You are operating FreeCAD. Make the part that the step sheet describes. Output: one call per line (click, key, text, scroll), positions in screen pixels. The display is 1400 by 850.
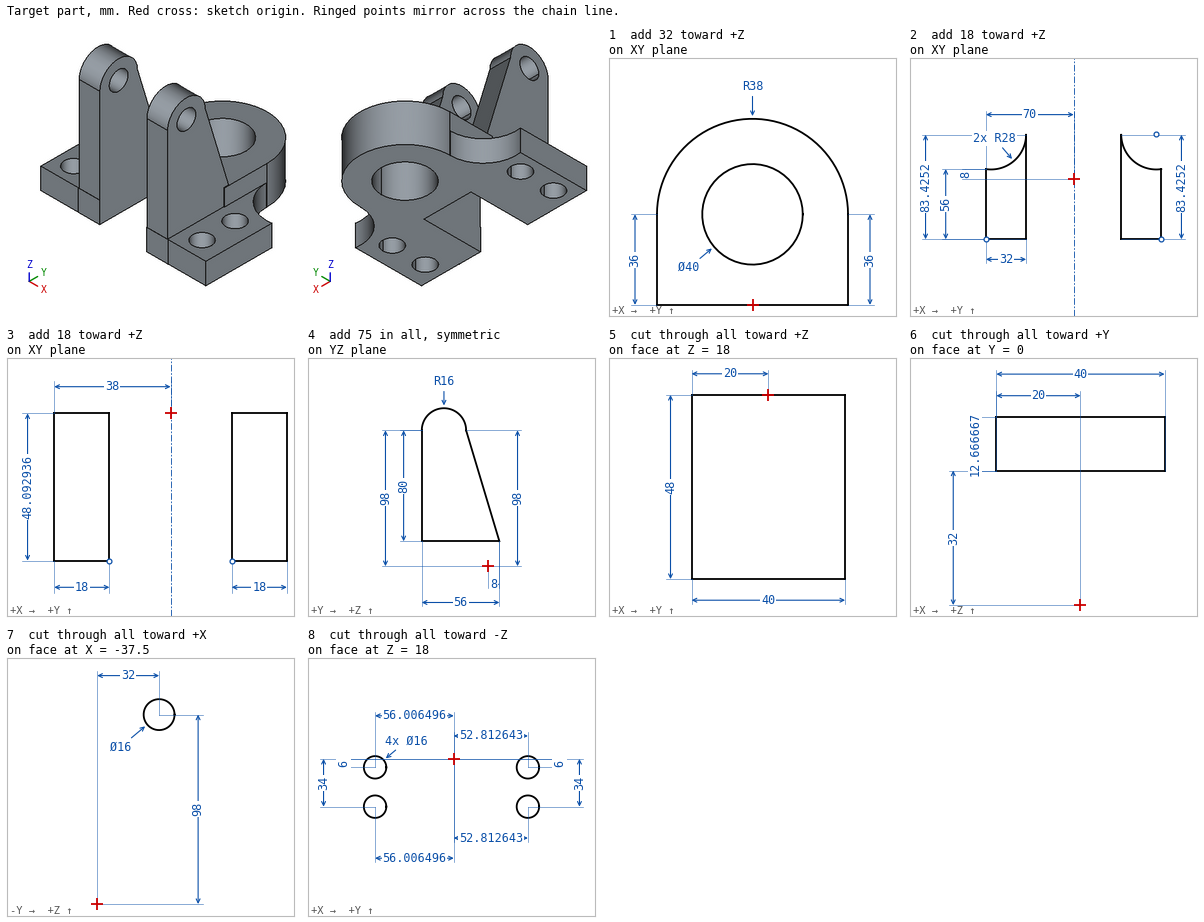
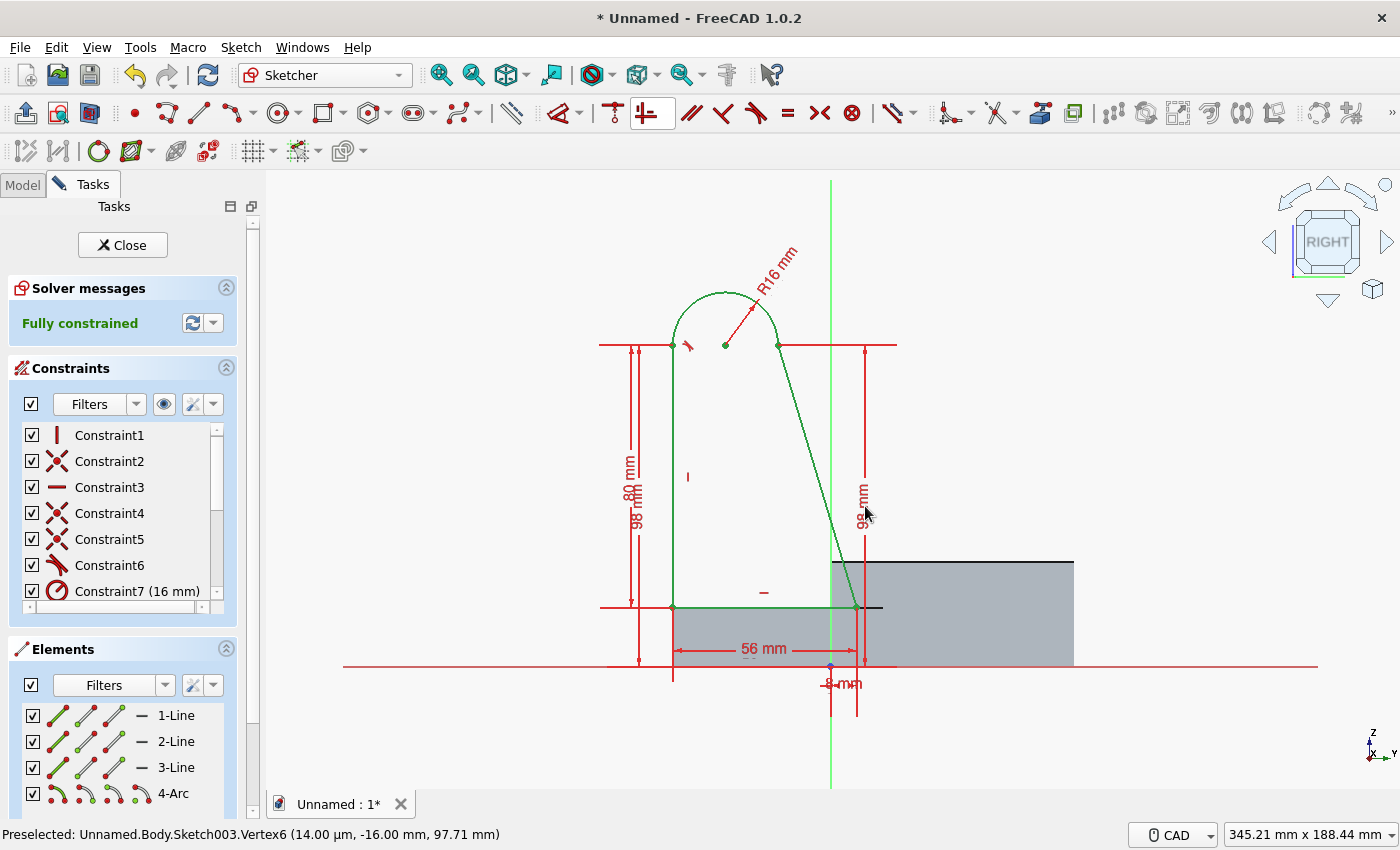
click(123, 245)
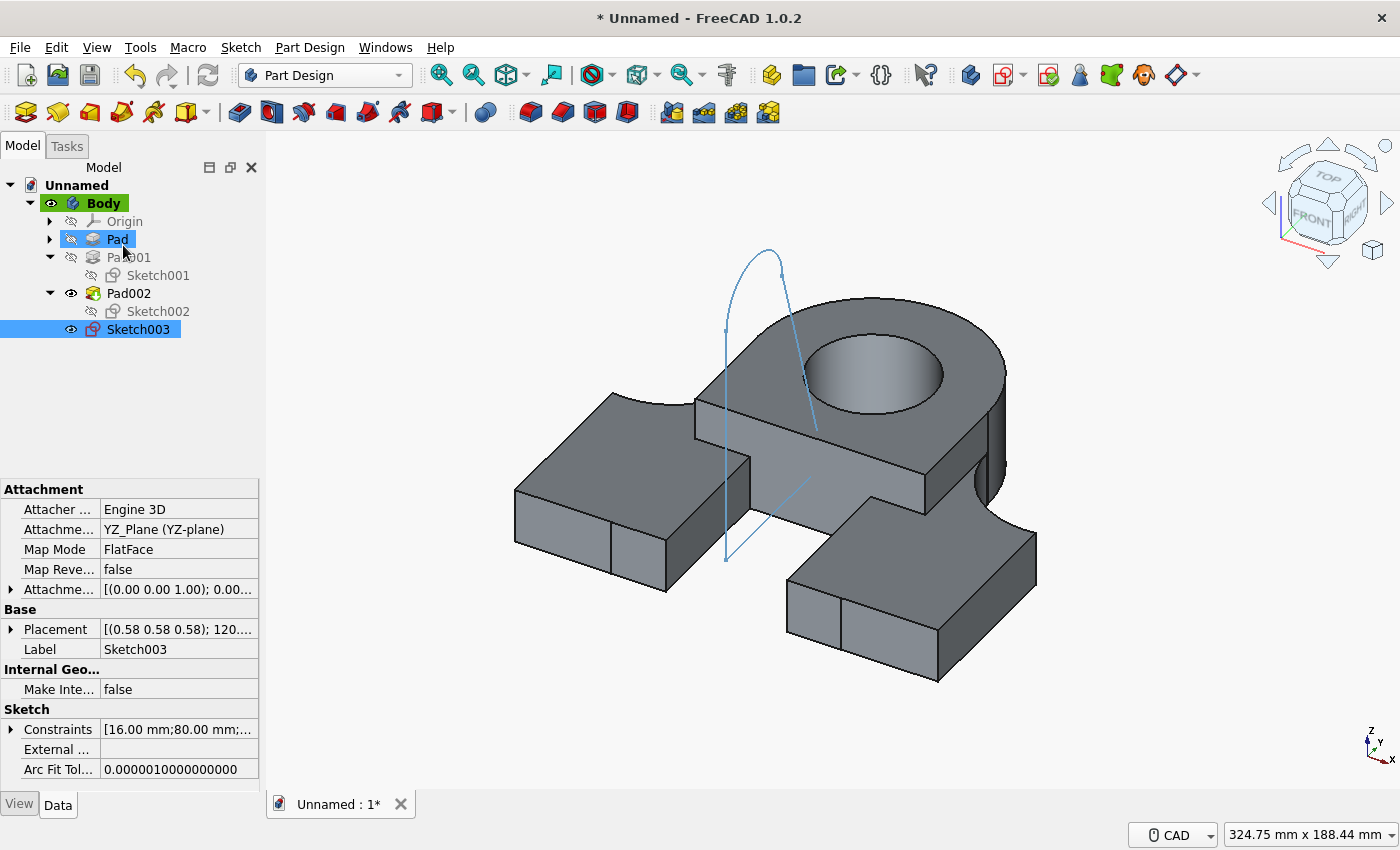
click(26, 112)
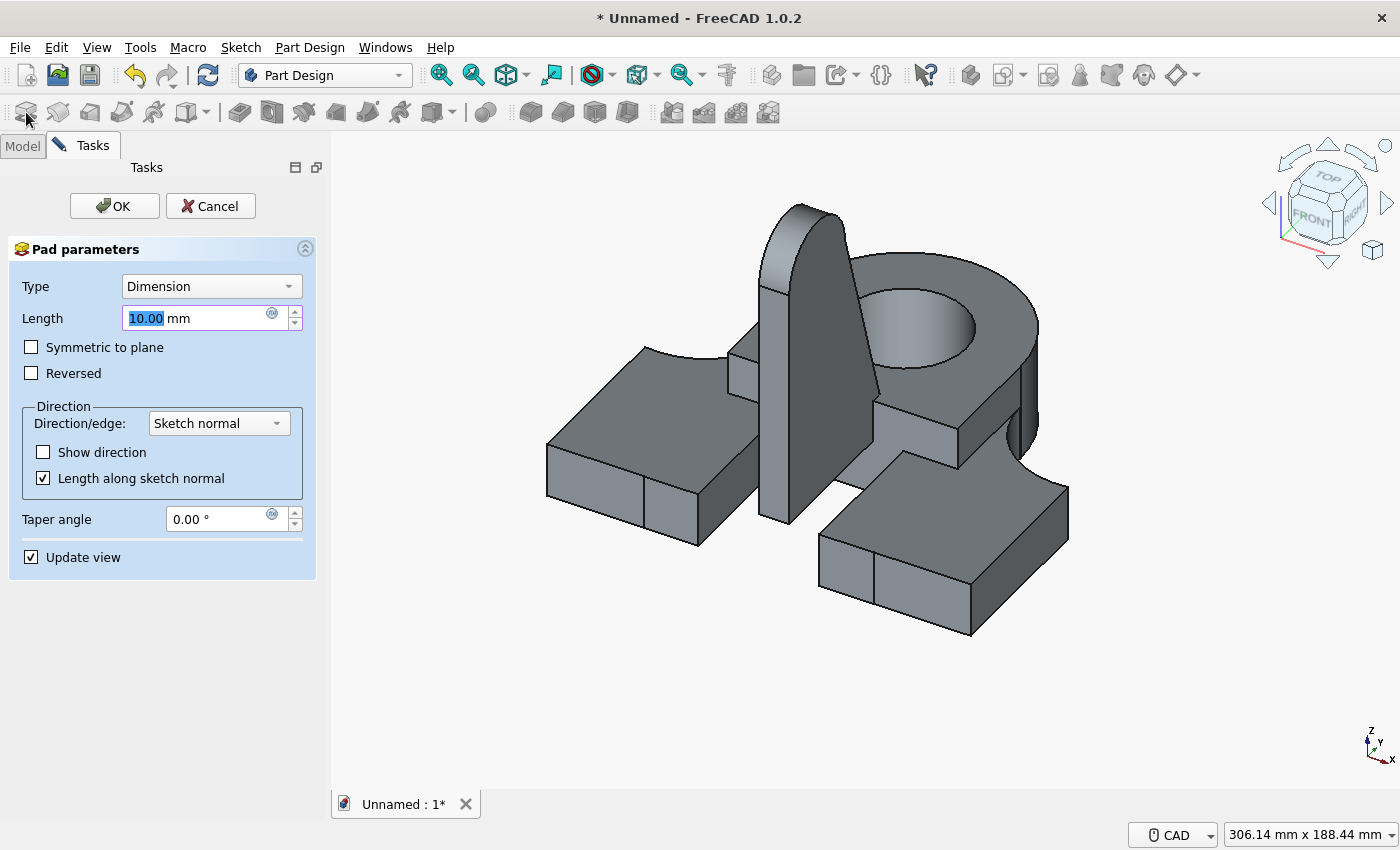
text(75)
key(Tab)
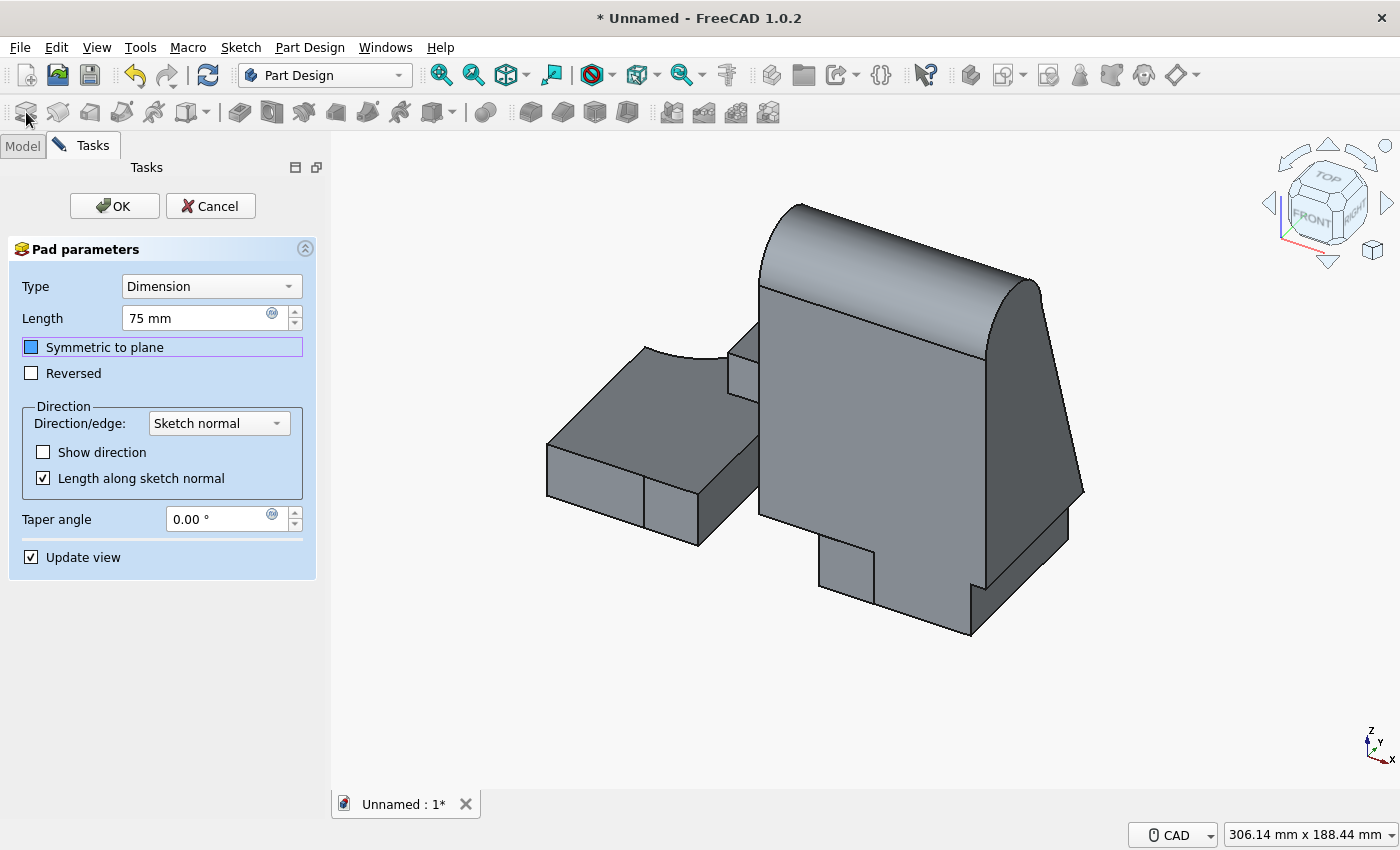
click(30, 347)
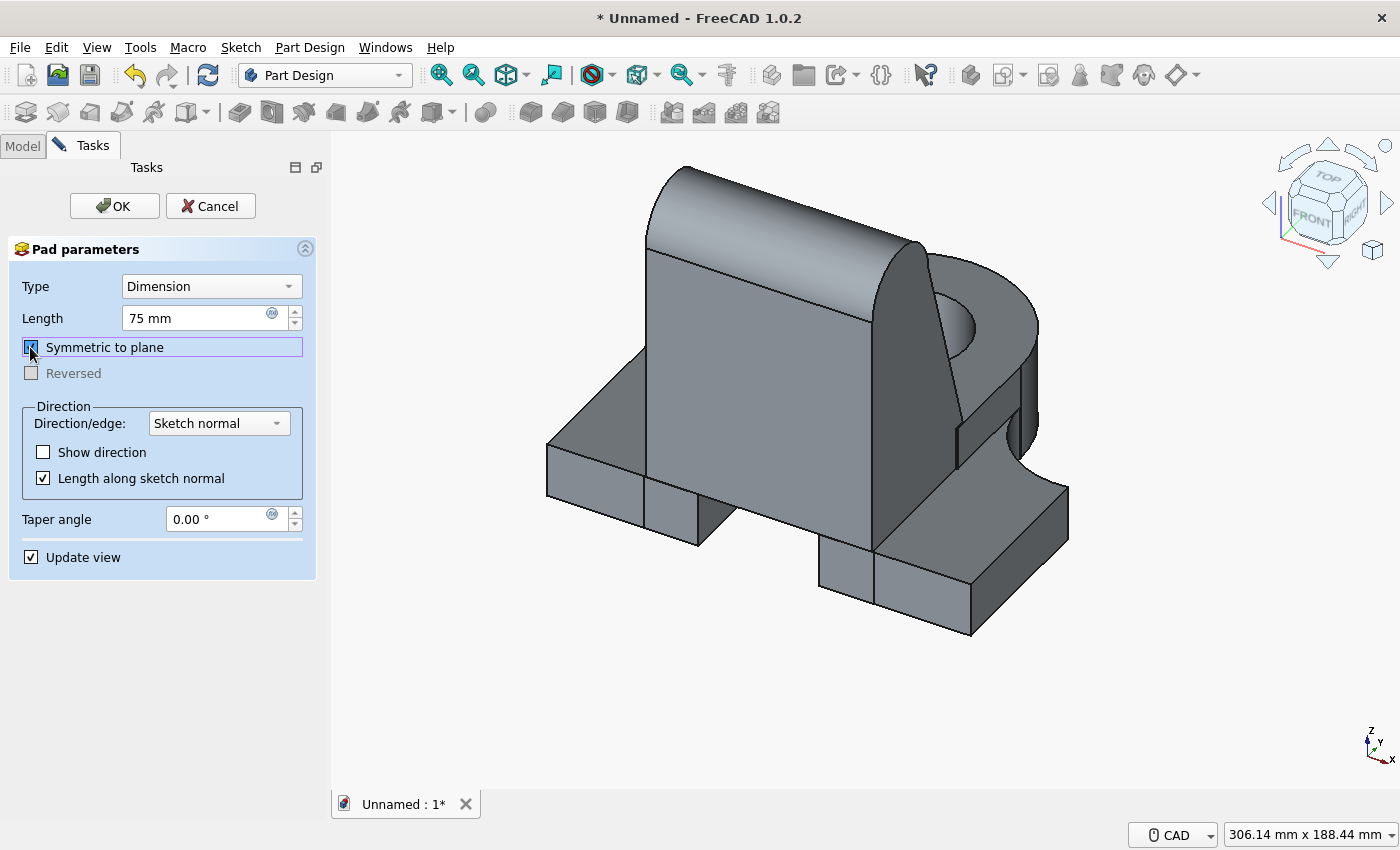
click(115, 206)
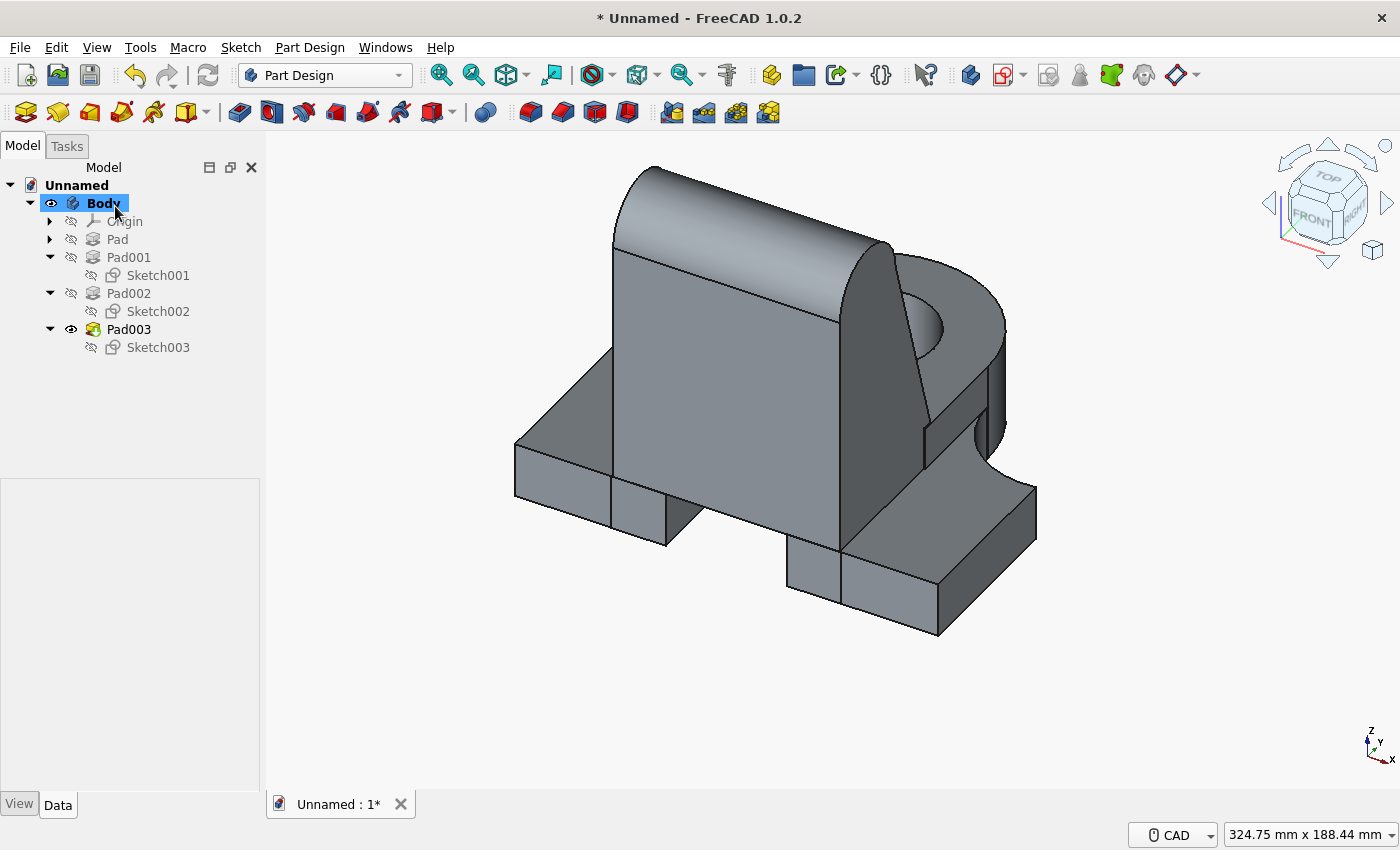
click(442, 76)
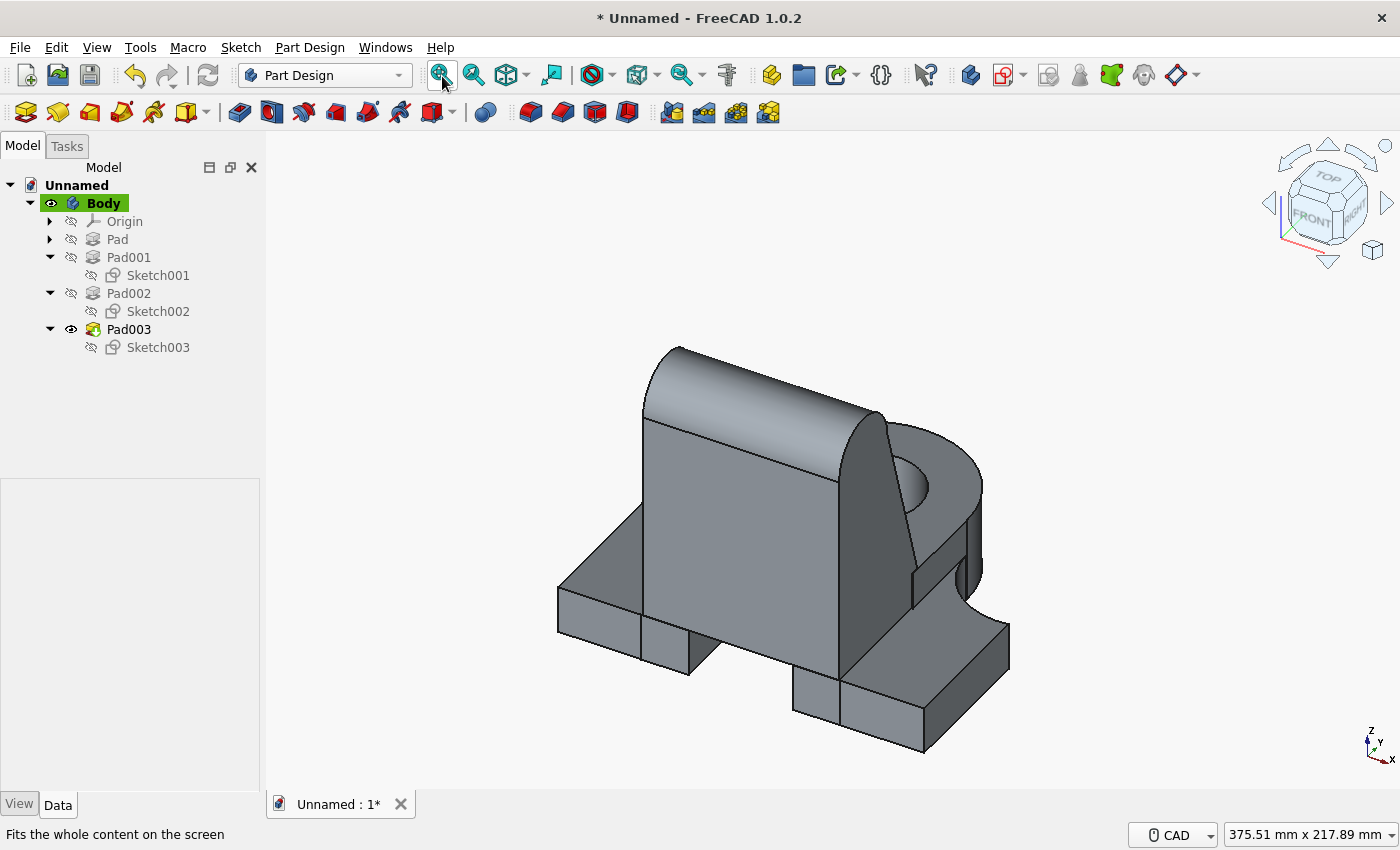
click(631, 575)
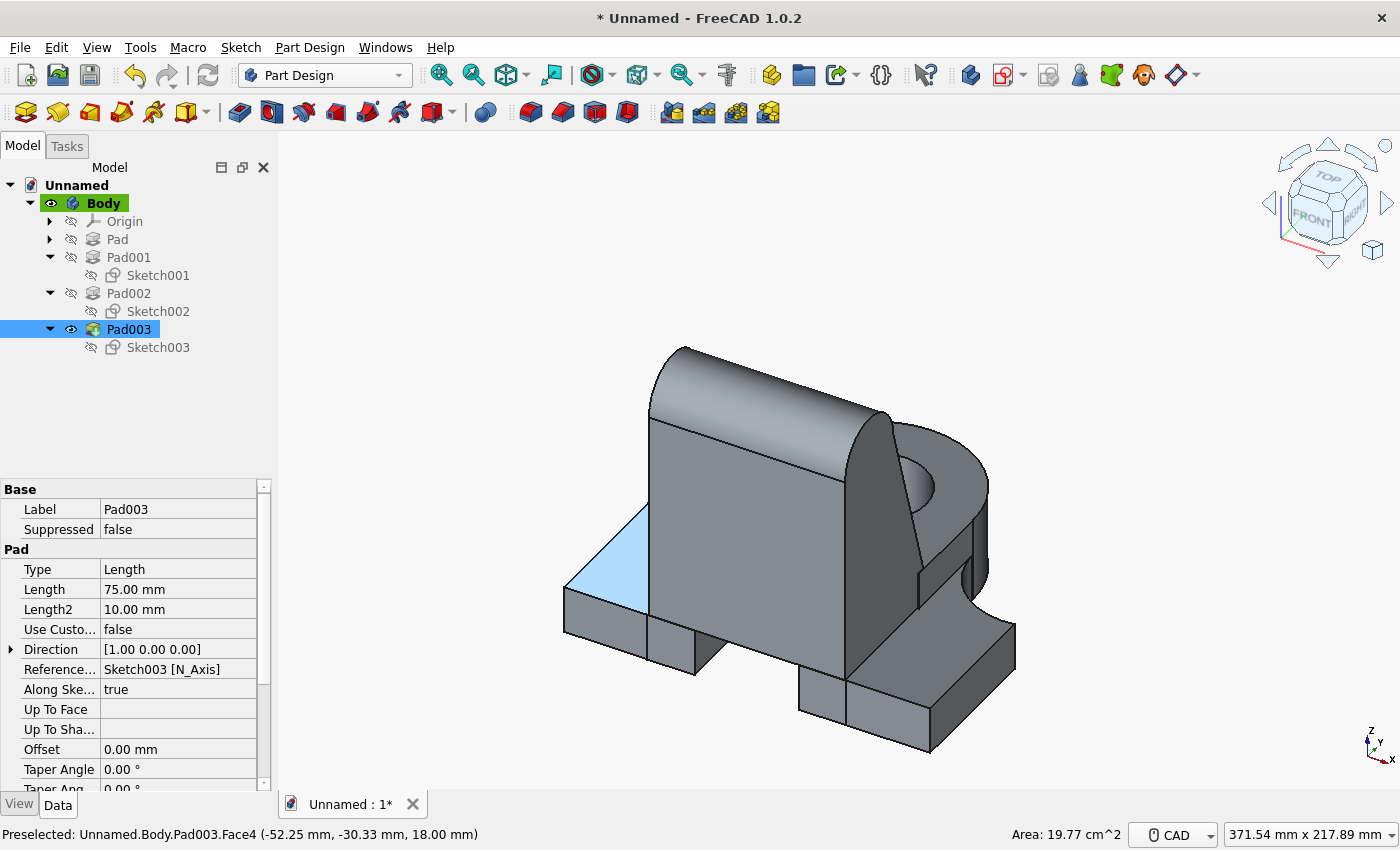
click(1004, 76)